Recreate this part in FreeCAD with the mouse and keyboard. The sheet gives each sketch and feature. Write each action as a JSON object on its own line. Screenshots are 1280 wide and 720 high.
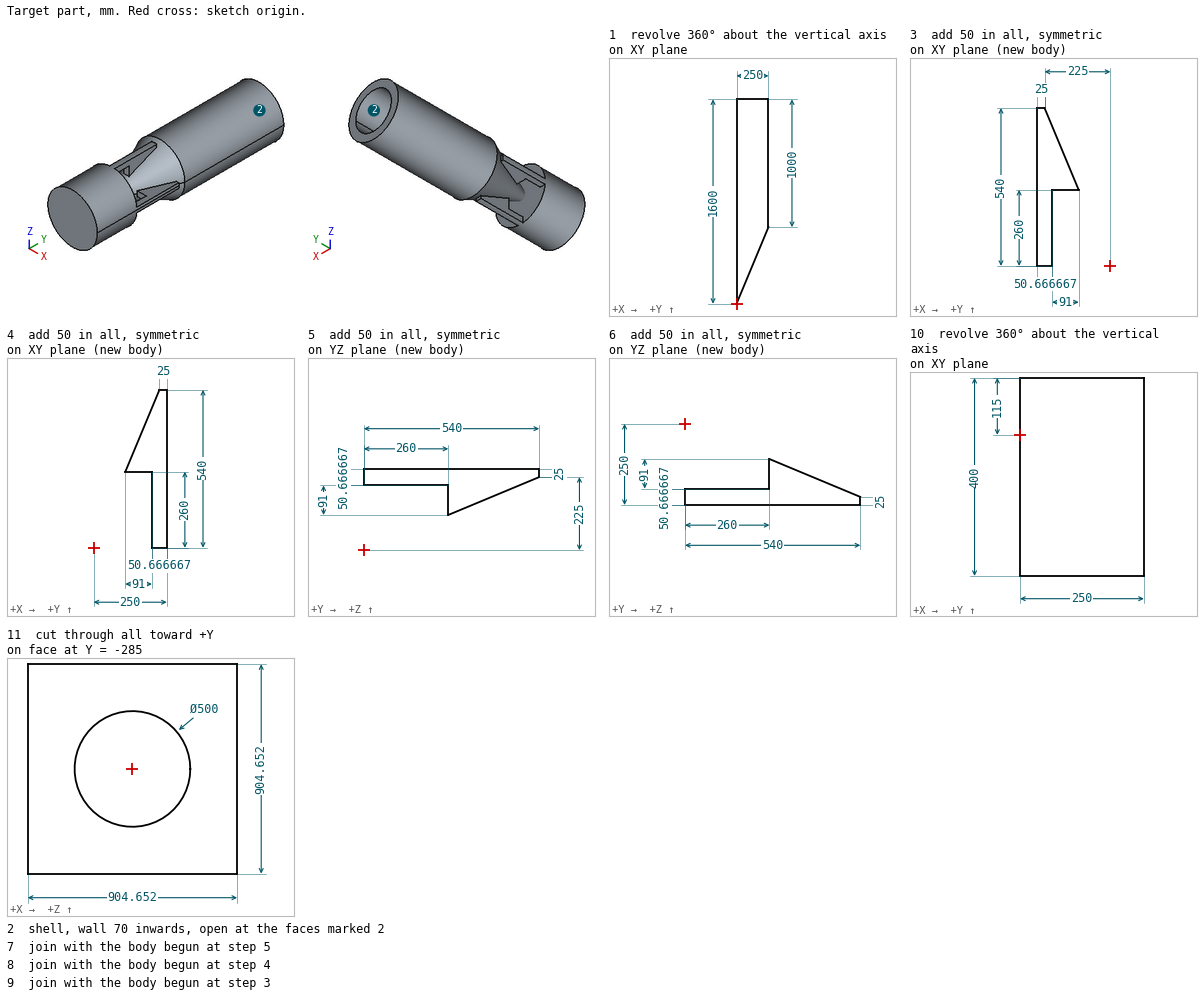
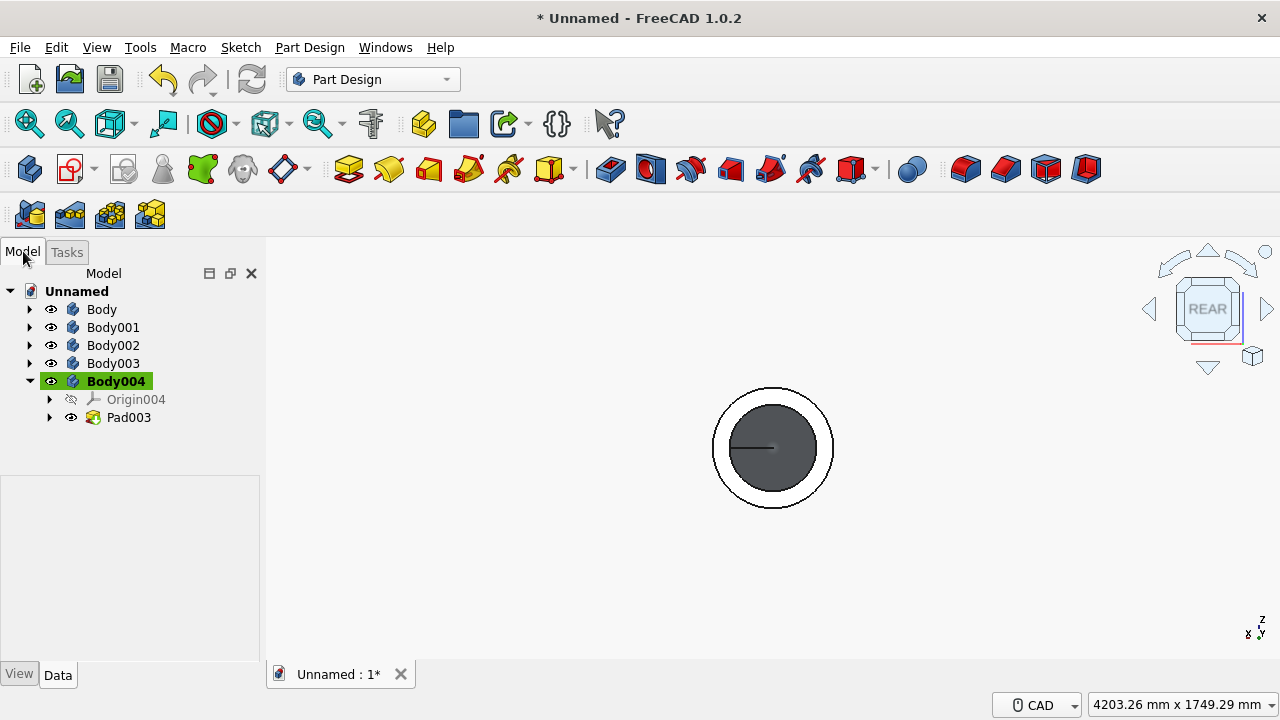
{"action": "left_click", "coordinate": [96, 381]}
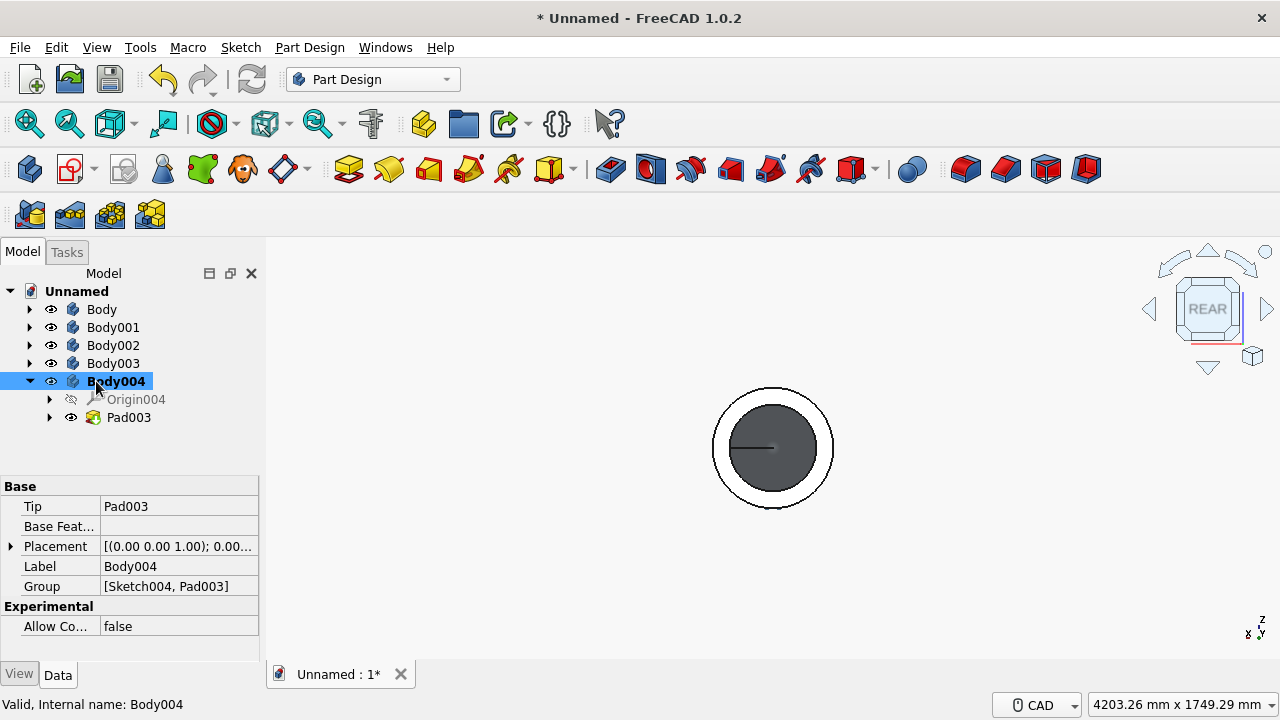
{"action": "left_click", "coordinate": [146, 626]}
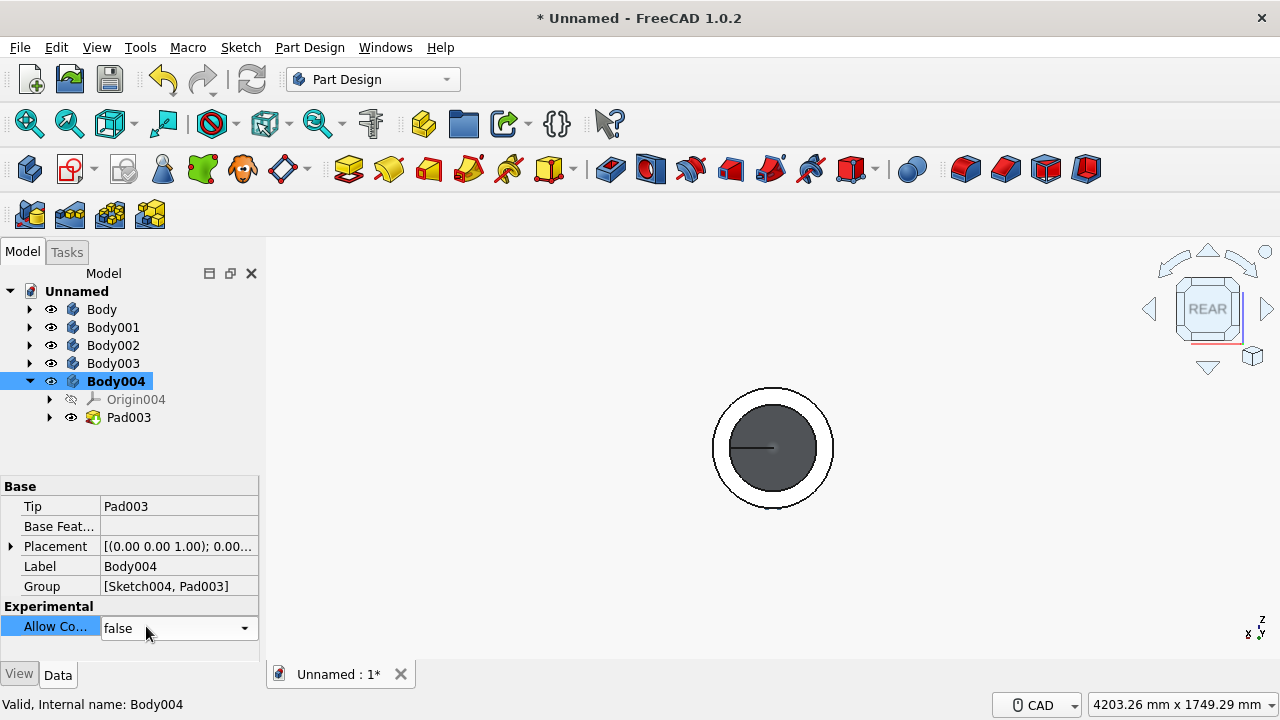
{"action": "left_click", "coordinate": [146, 626]}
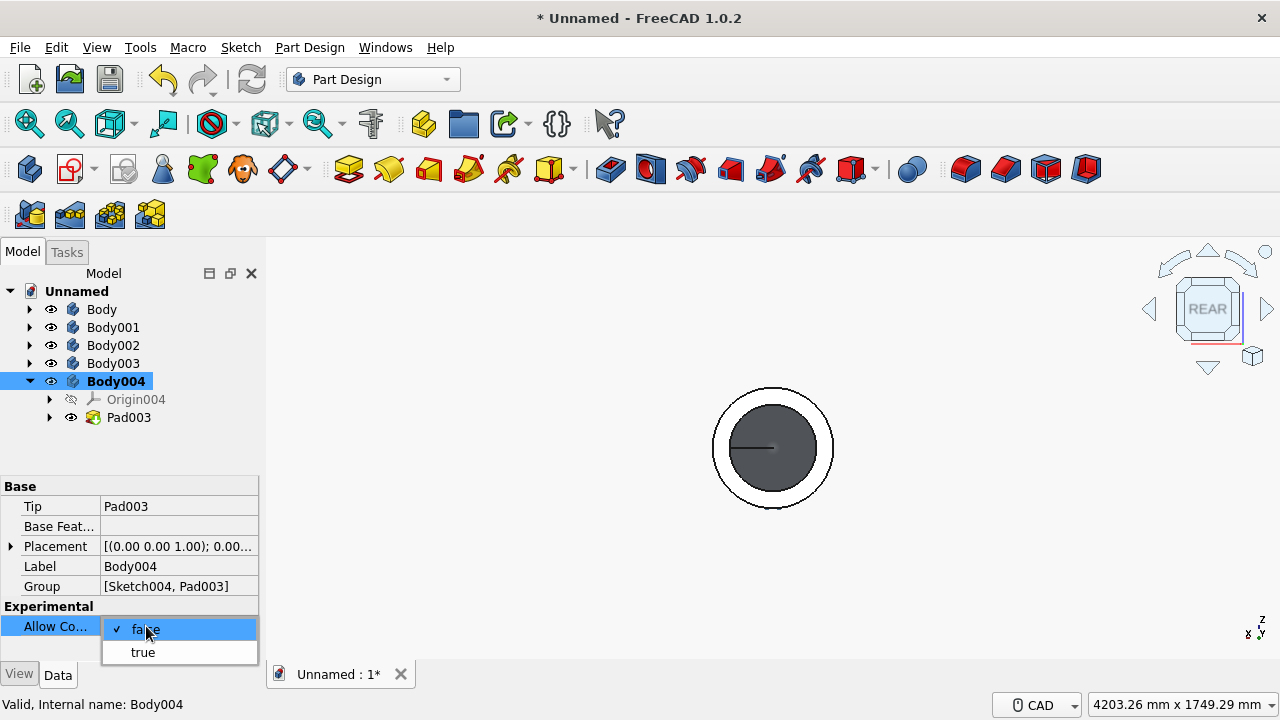
{"action": "left_click", "coordinate": [179, 652]}
{"action": "key", "text": "Return"}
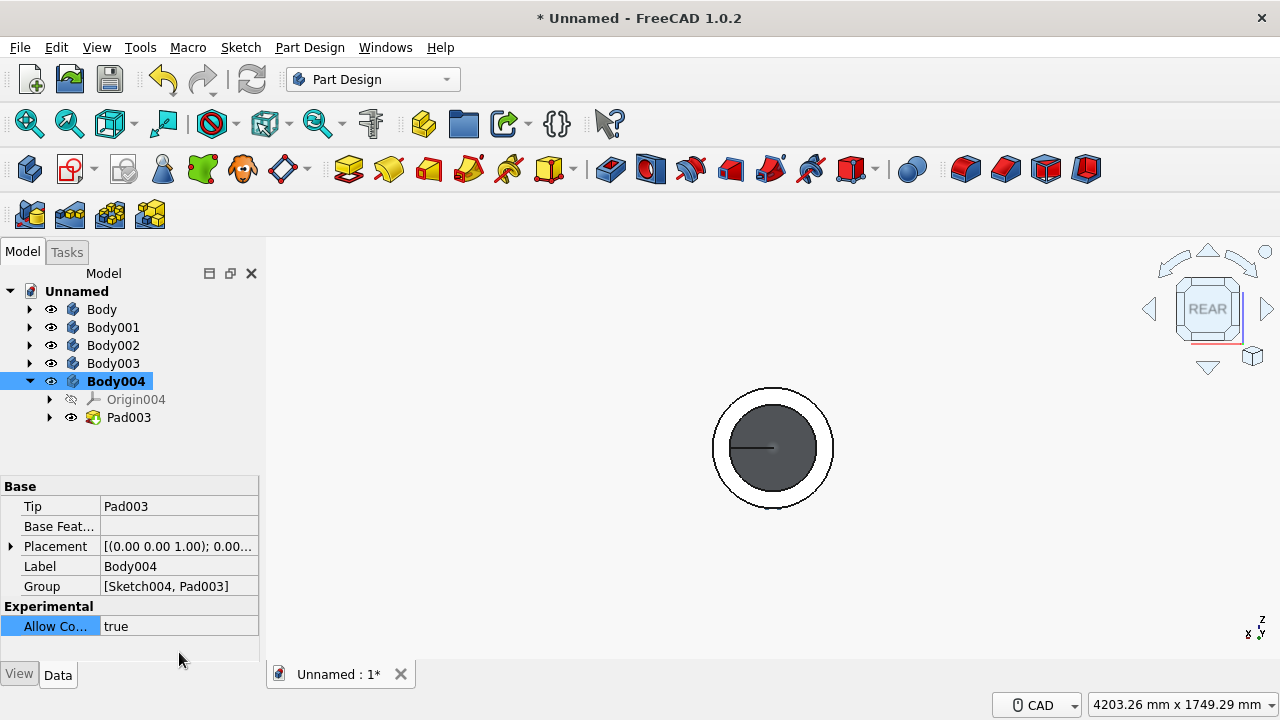
{"action": "left_click", "coordinate": [96, 363]}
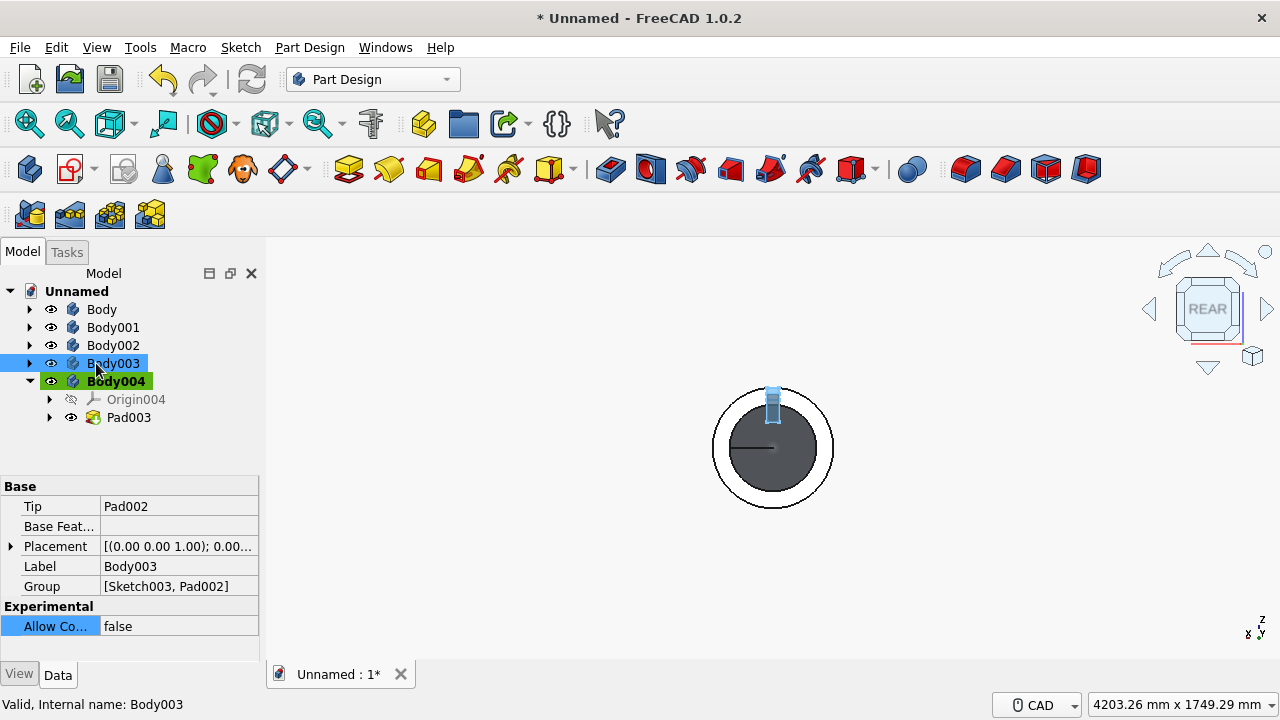
{"action": "left_click", "coordinate": [914, 170]}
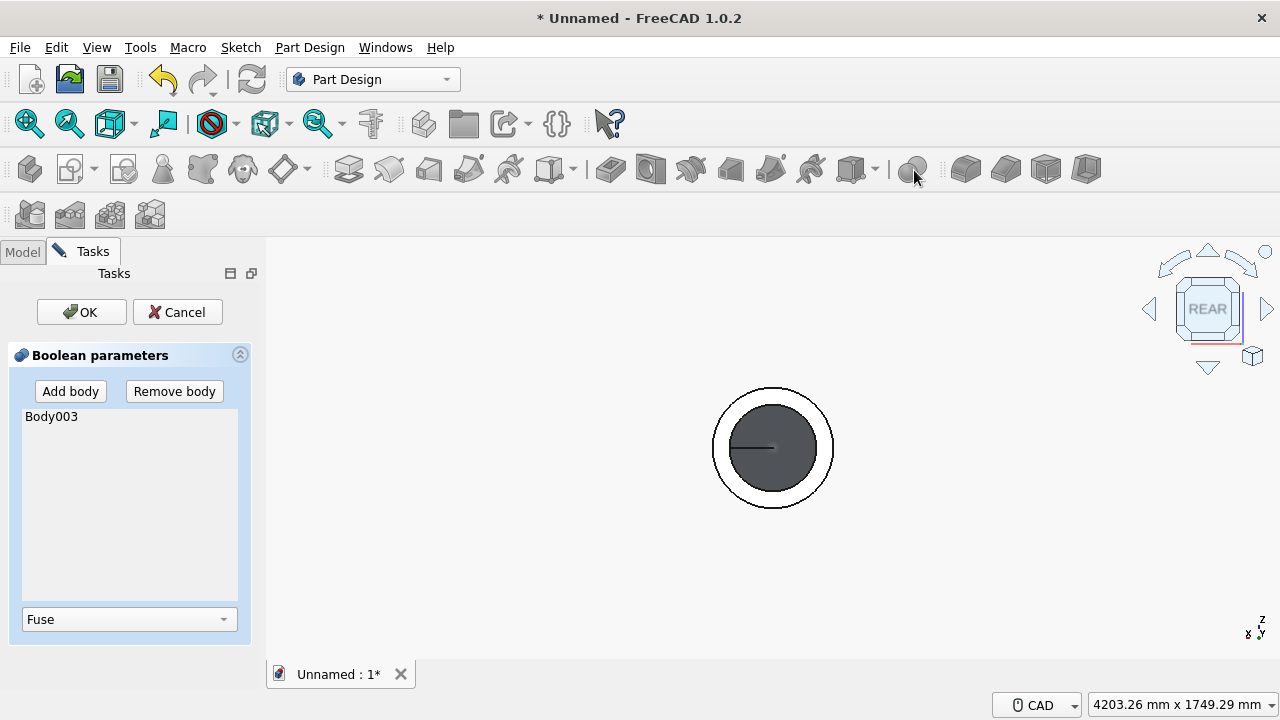
{"action": "left_click", "coordinate": [82, 312]}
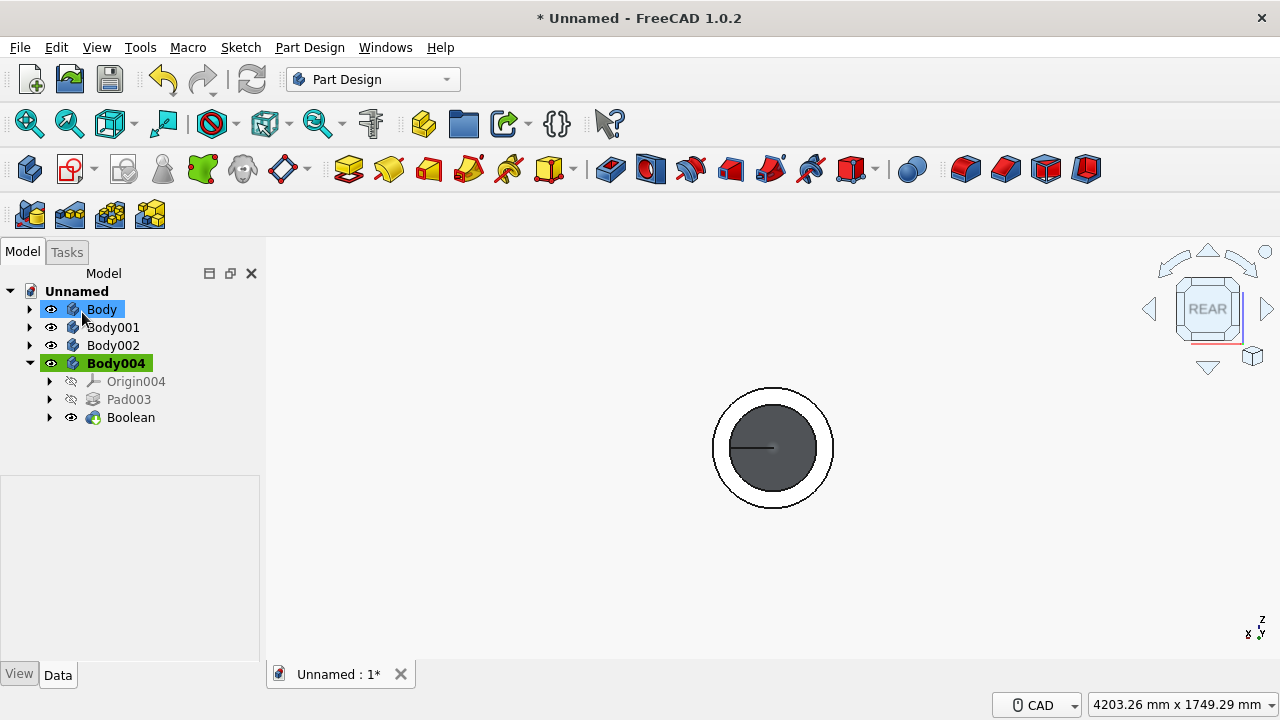
{"action": "left_click", "coordinate": [30, 124]}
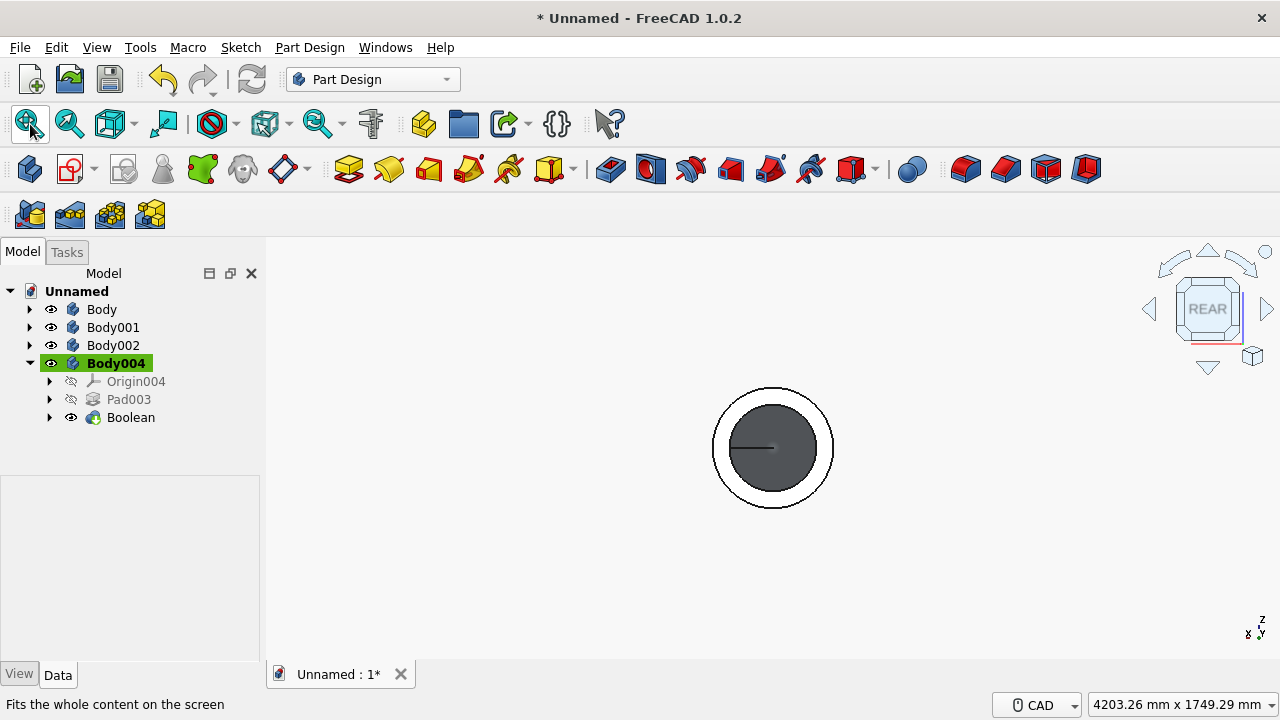
{"action": "left_click", "coordinate": [96, 345]}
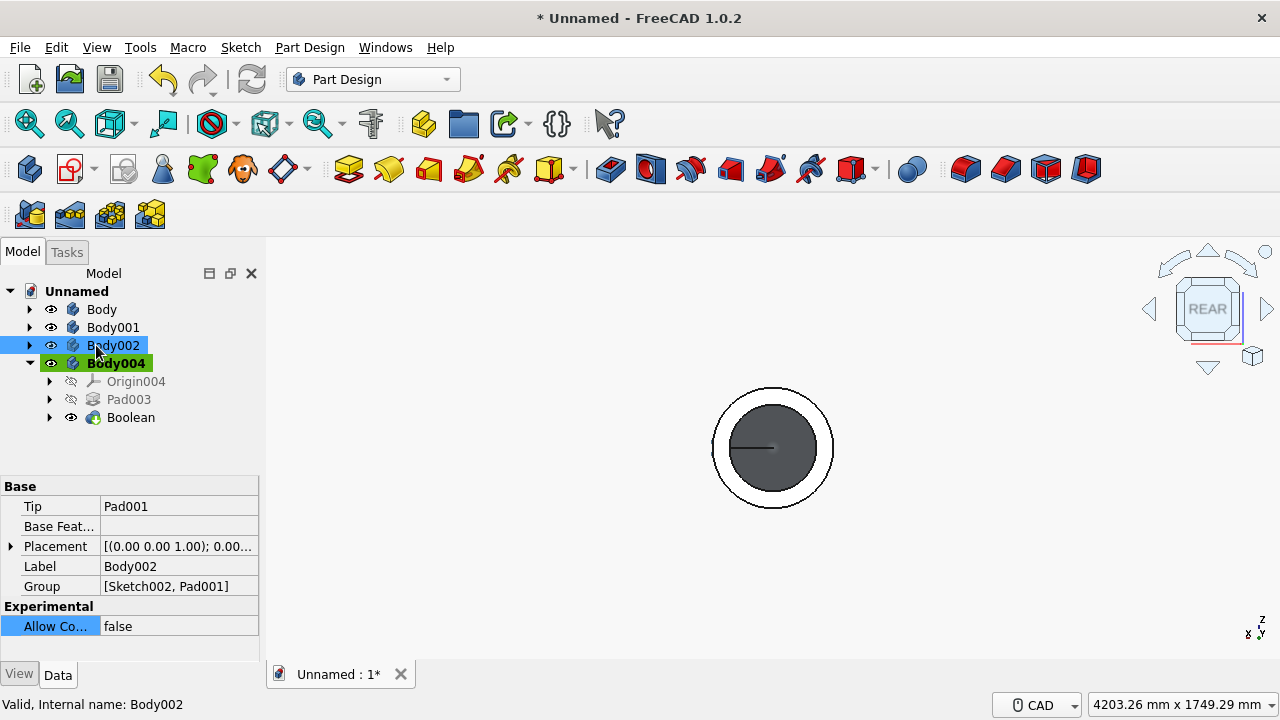
{"action": "left_click", "coordinate": [914, 170]}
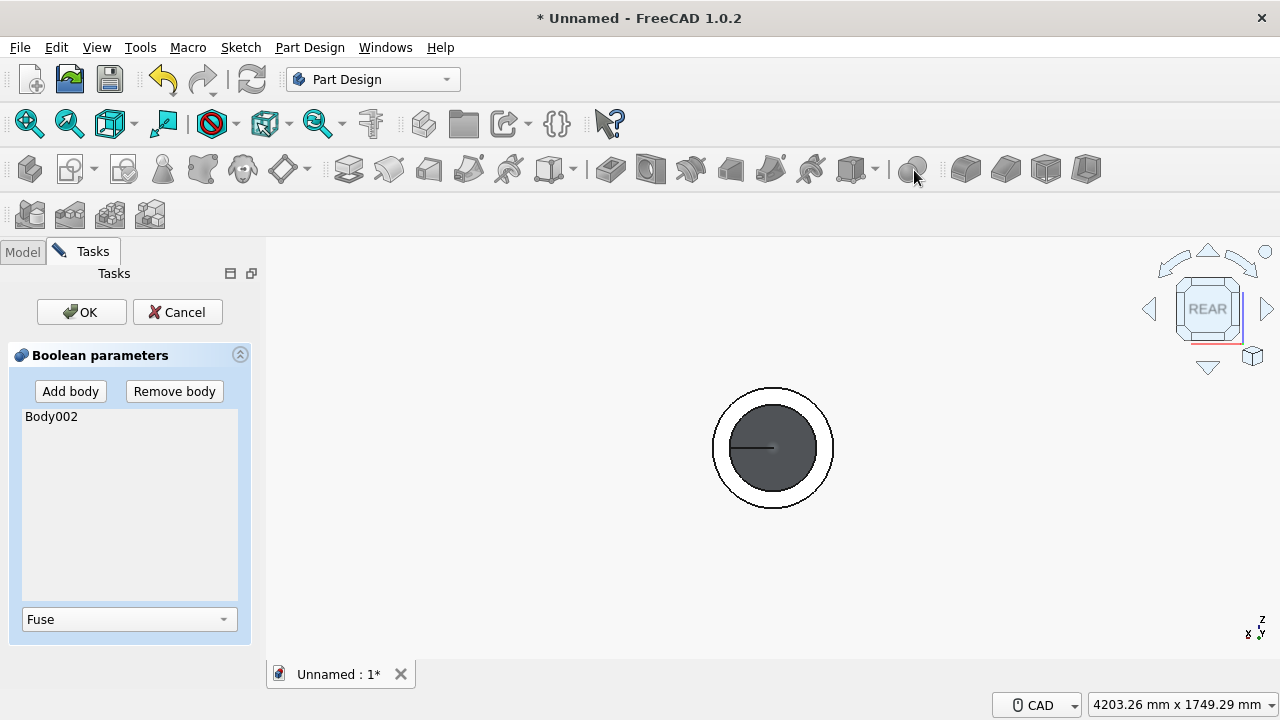
{"action": "left_click", "coordinate": [82, 312]}